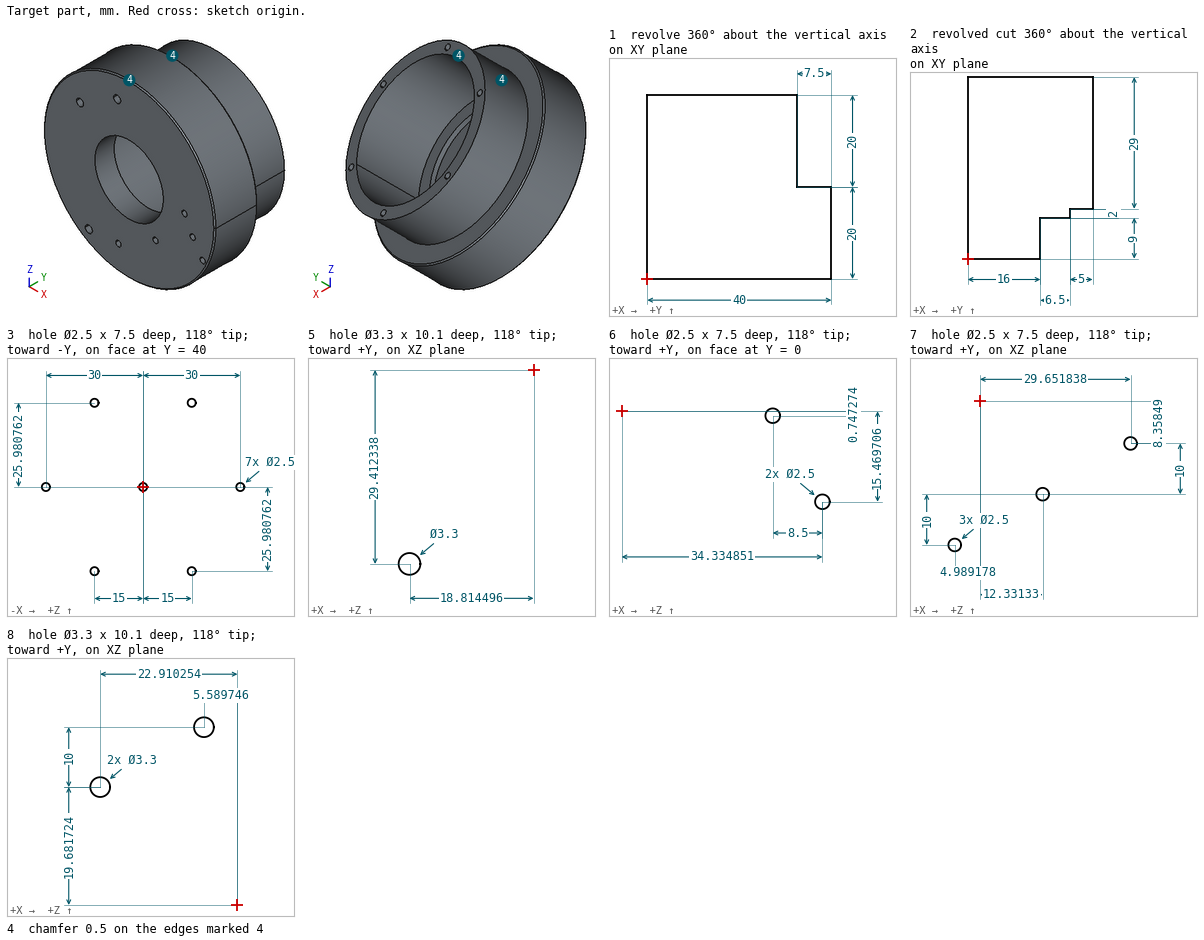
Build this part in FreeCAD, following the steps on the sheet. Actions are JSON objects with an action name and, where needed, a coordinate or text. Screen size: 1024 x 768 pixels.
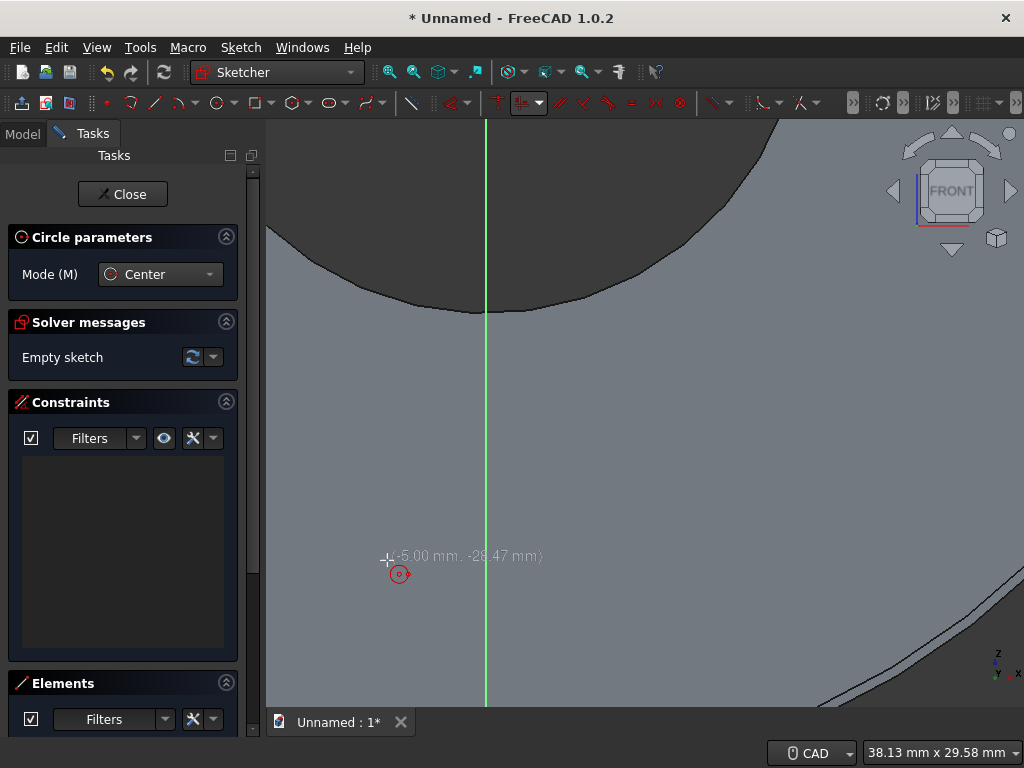
{"action": "left_click", "coordinate": [387, 559]}
{"action": "mouse_move", "coordinate": [405, 541]}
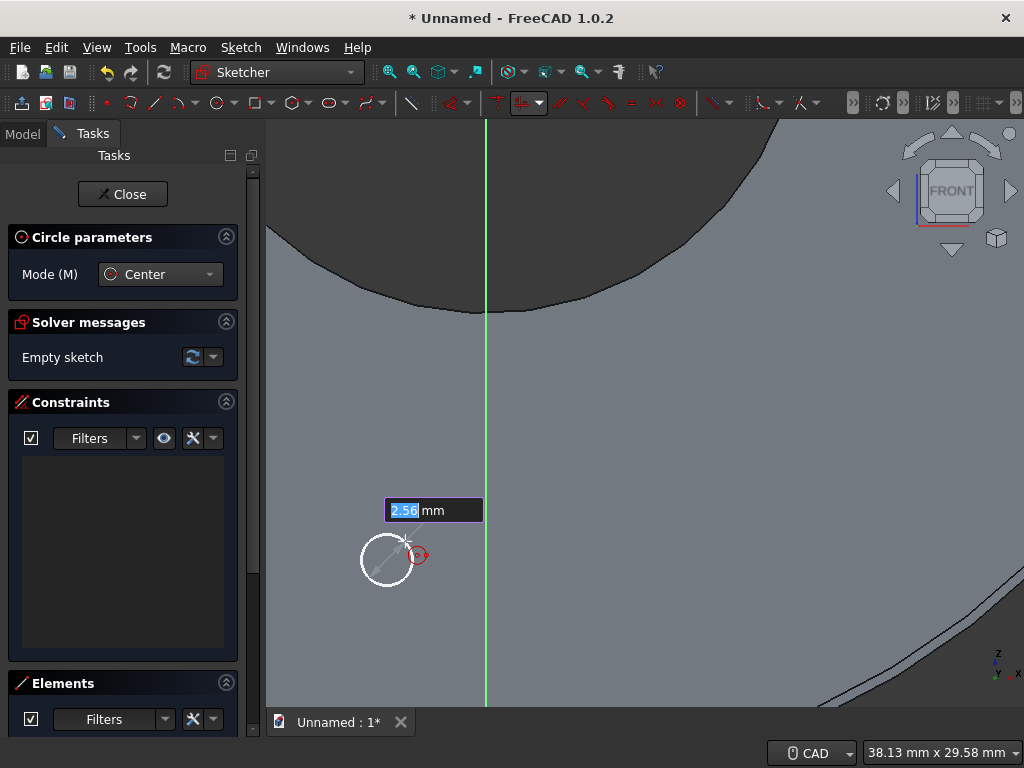
{"action": "type", "text": "2.5"}
{"action": "key", "text": "Return"}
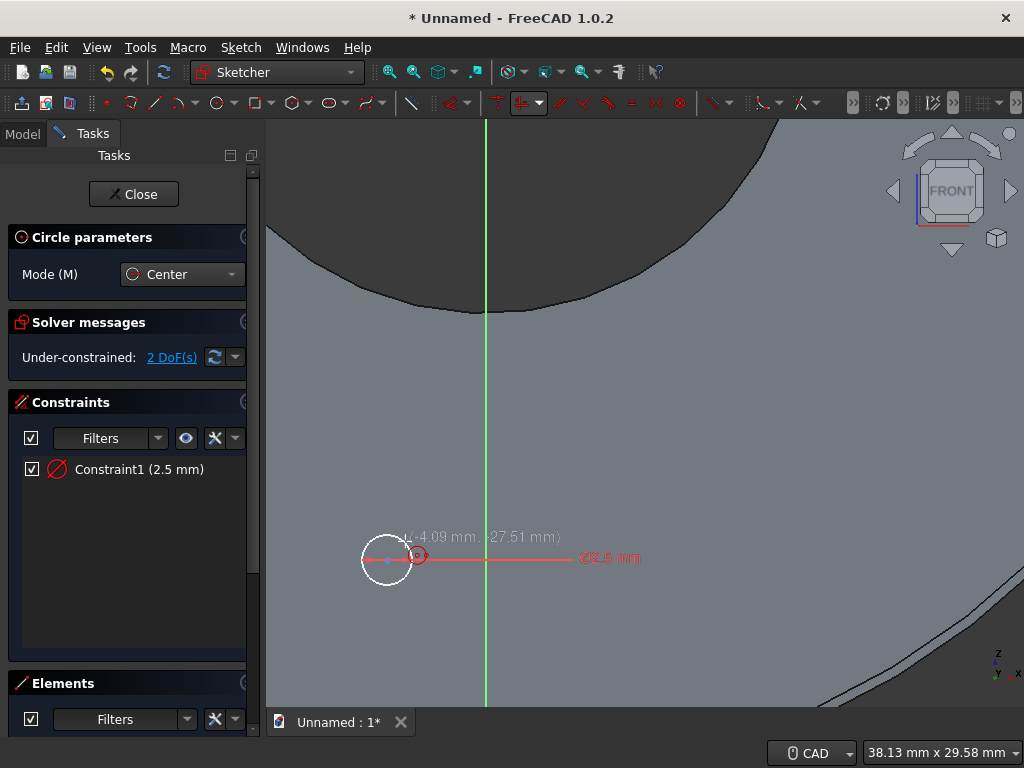
{"action": "left_click", "coordinate": [731, 360]}
{"action": "mouse_move", "coordinate": [749, 343]}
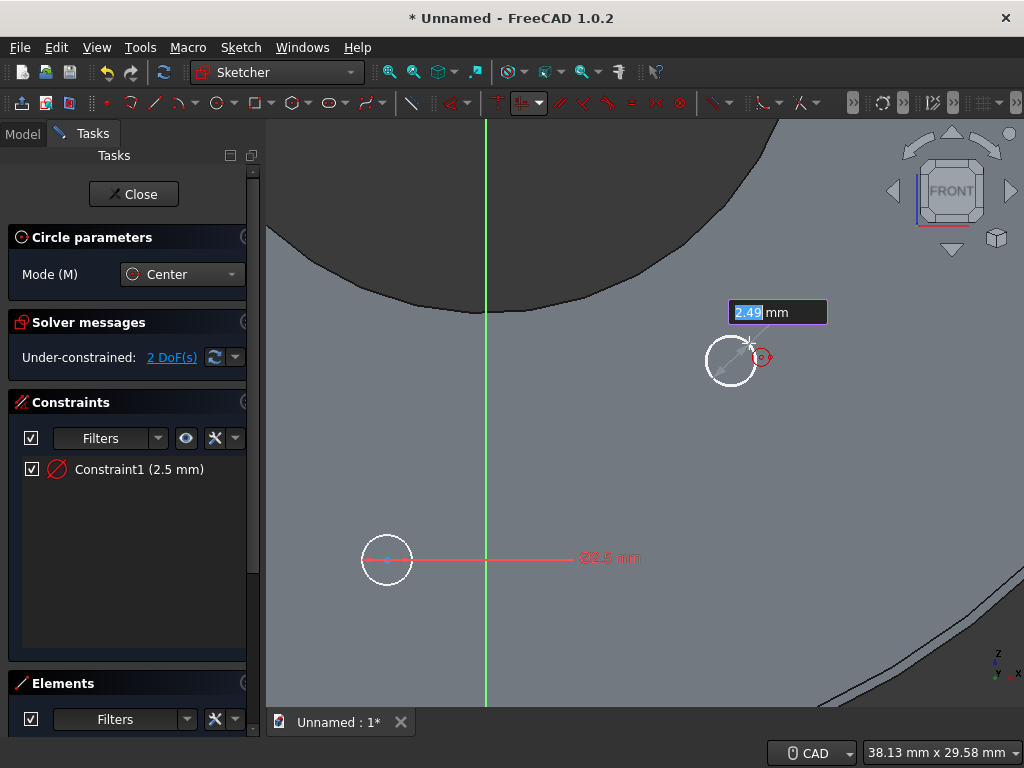
{"action": "type", "text": "2.5"}
{"action": "key", "text": "Return"}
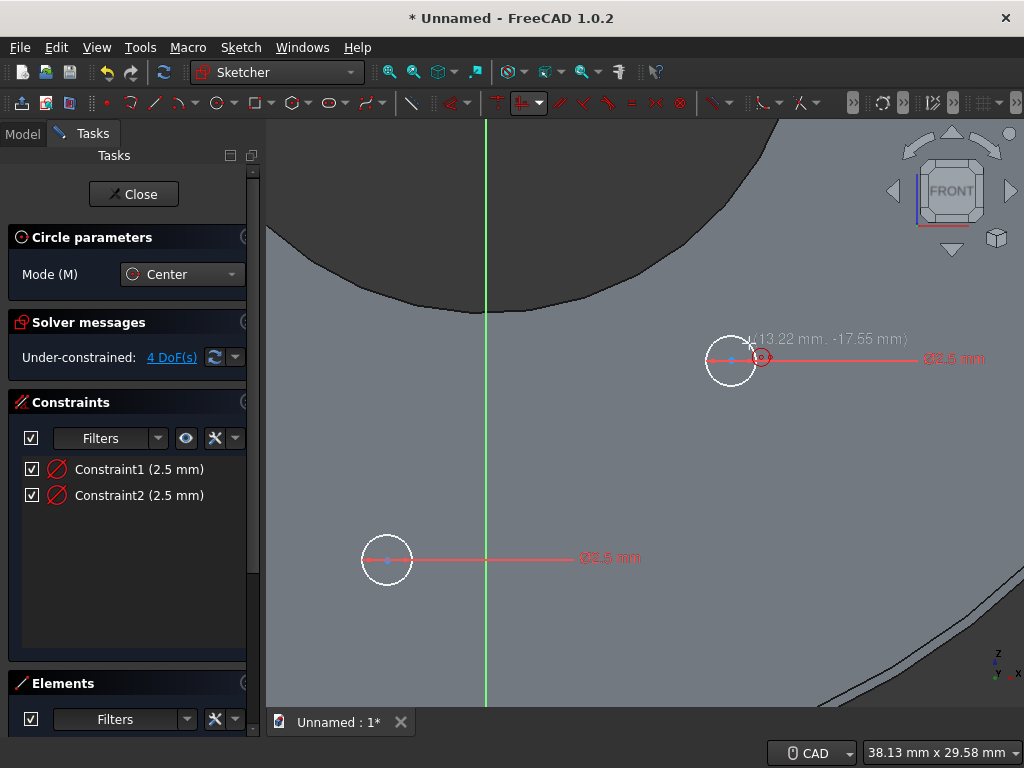
{"action": "scroll", "coordinate": [388, 563], "scroll_direction": "down", "scroll_amount": 3}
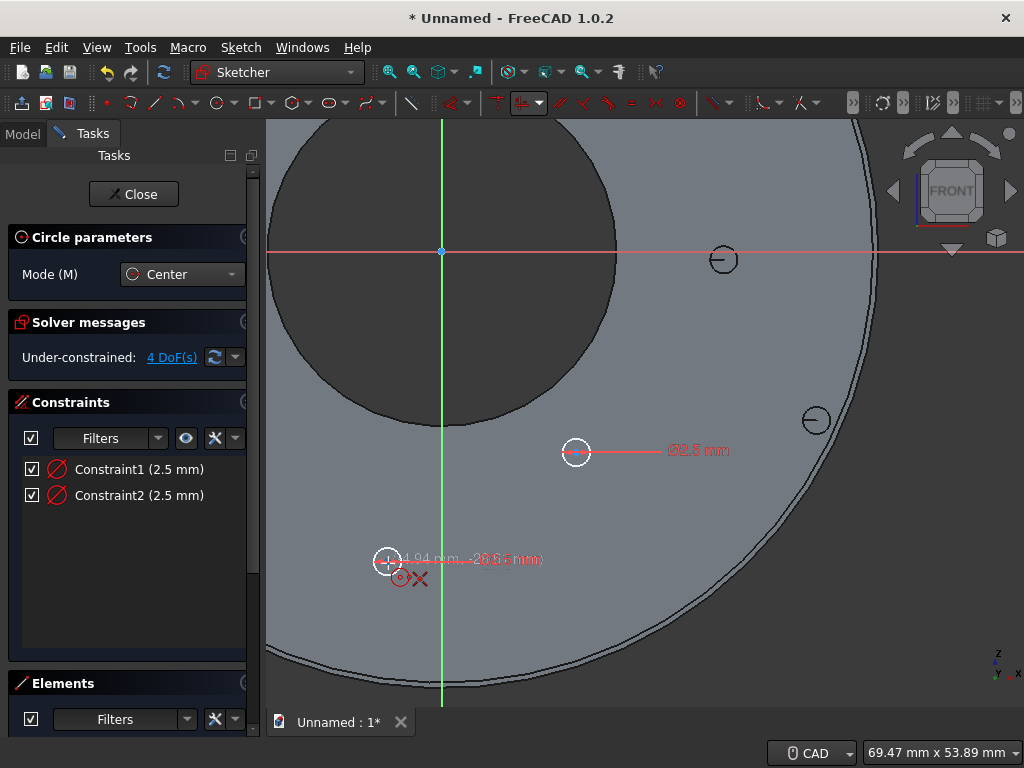
{"action": "scroll", "coordinate": [766, 343], "scroll_direction": "up", "scroll_amount": 3}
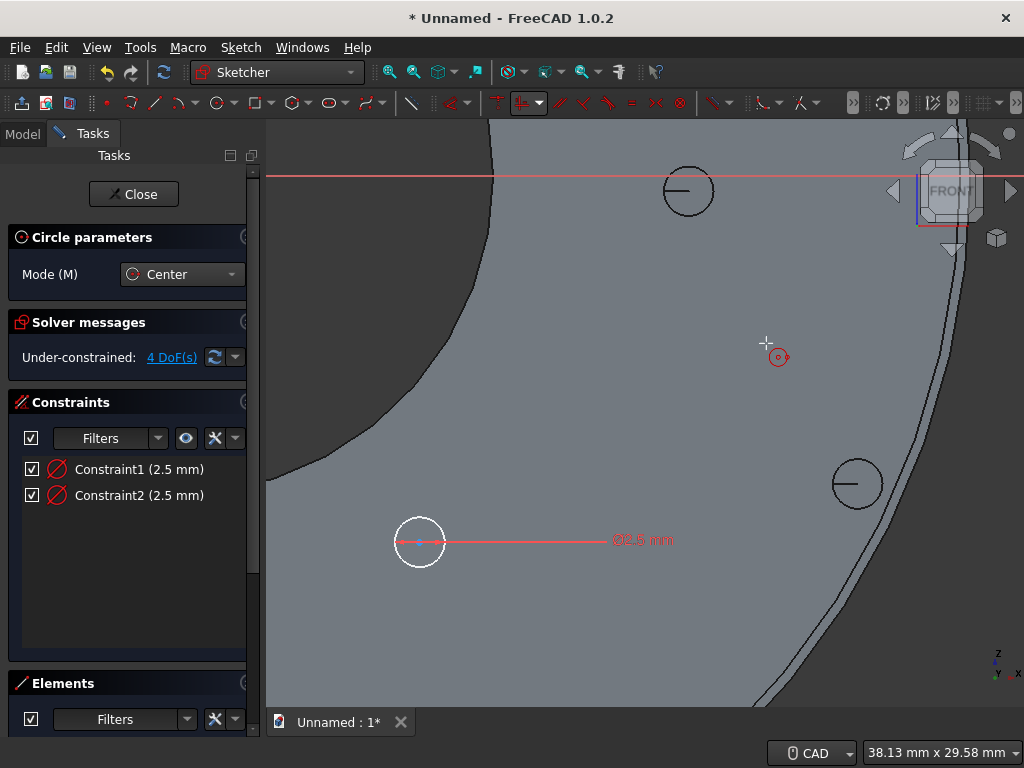
{"action": "left_click", "coordinate": [765, 343]}
{"action": "mouse_move", "coordinate": [782, 325]}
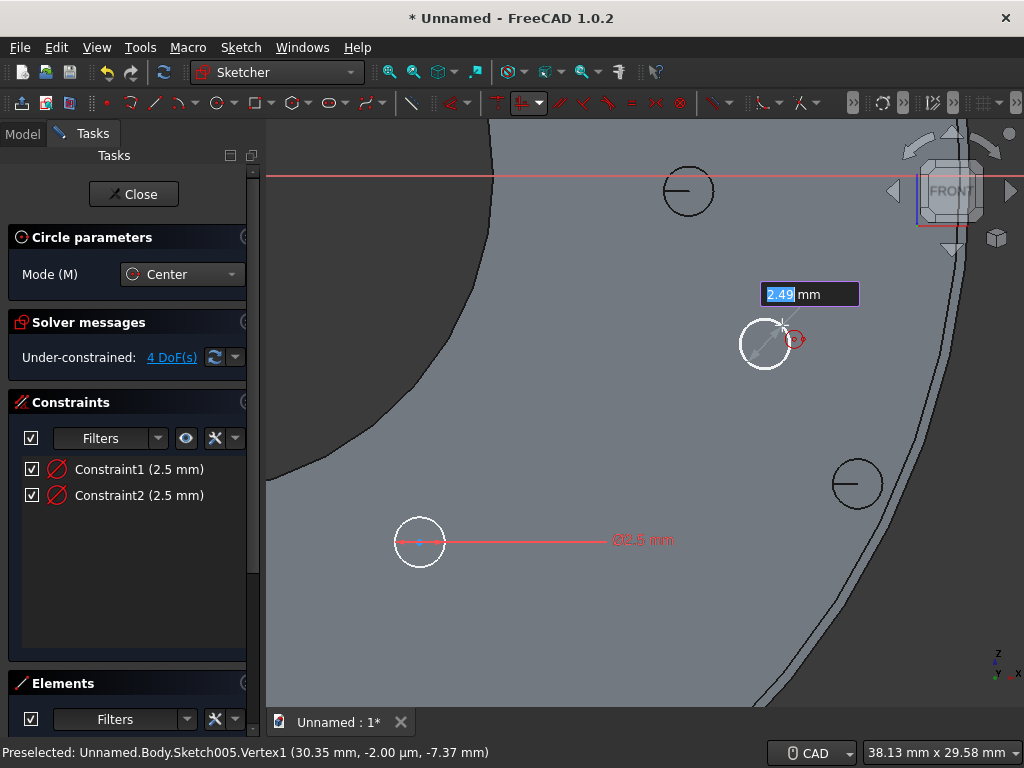
{"action": "type", "text": "2.5"}
{"action": "key", "text": "Return"}
{"action": "key", "text": "Escape"}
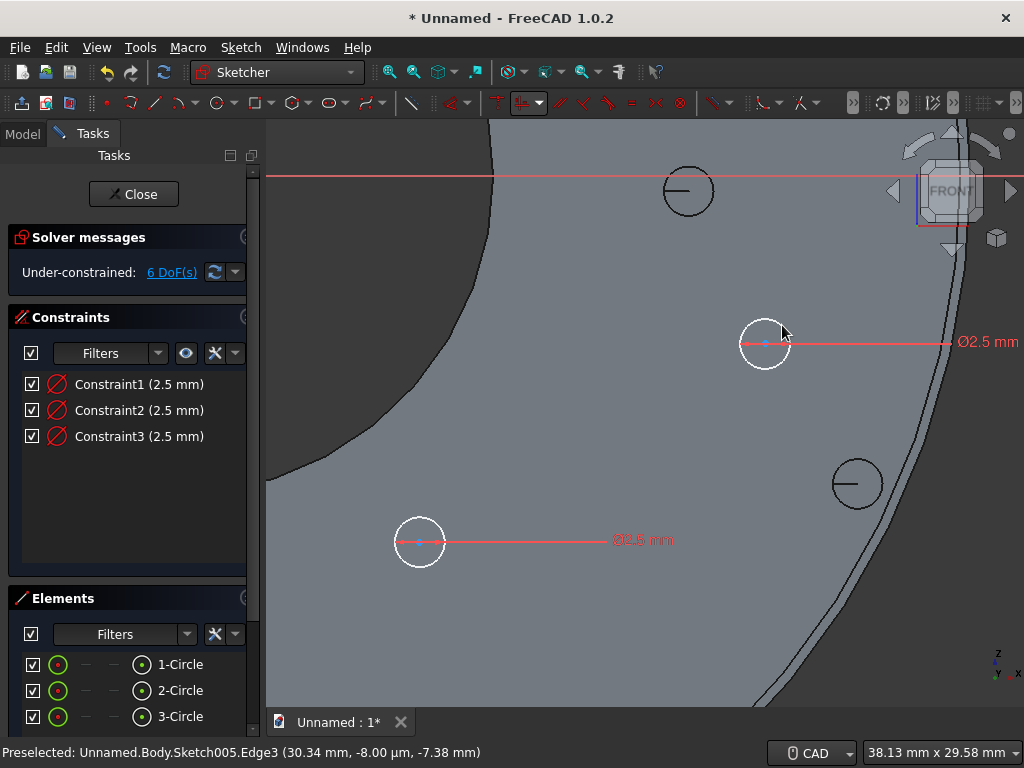
{"action": "left_click", "coordinate": [450, 104]}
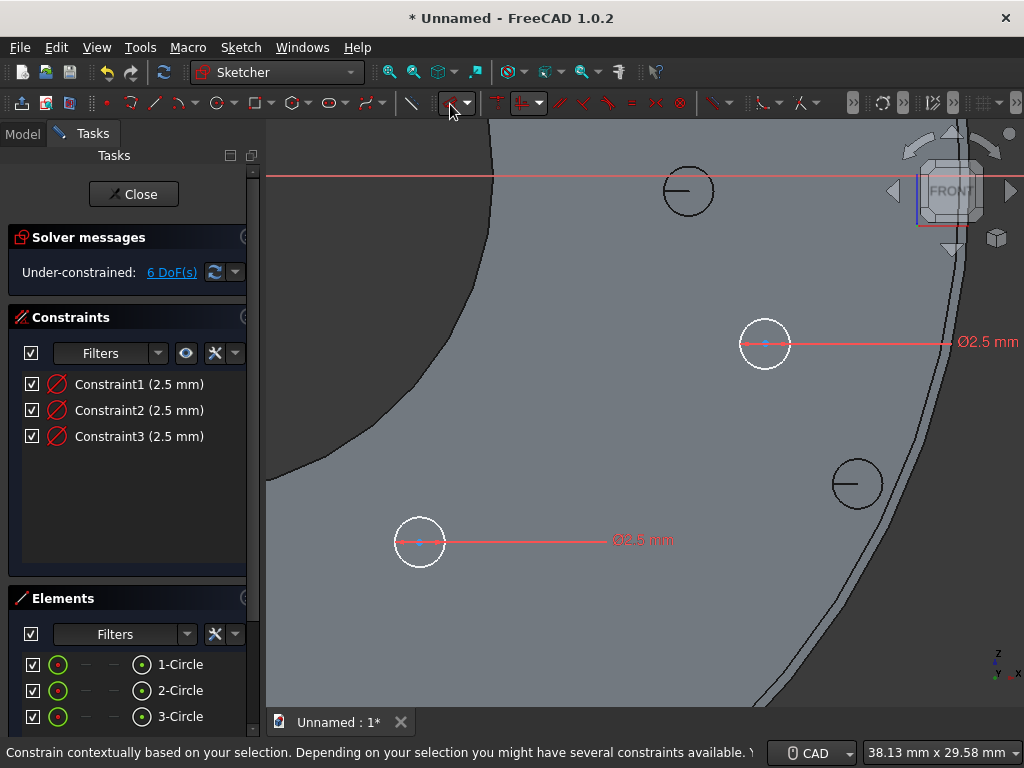
{"action": "scroll", "coordinate": [767, 343], "scroll_direction": "down", "scroll_amount": 3}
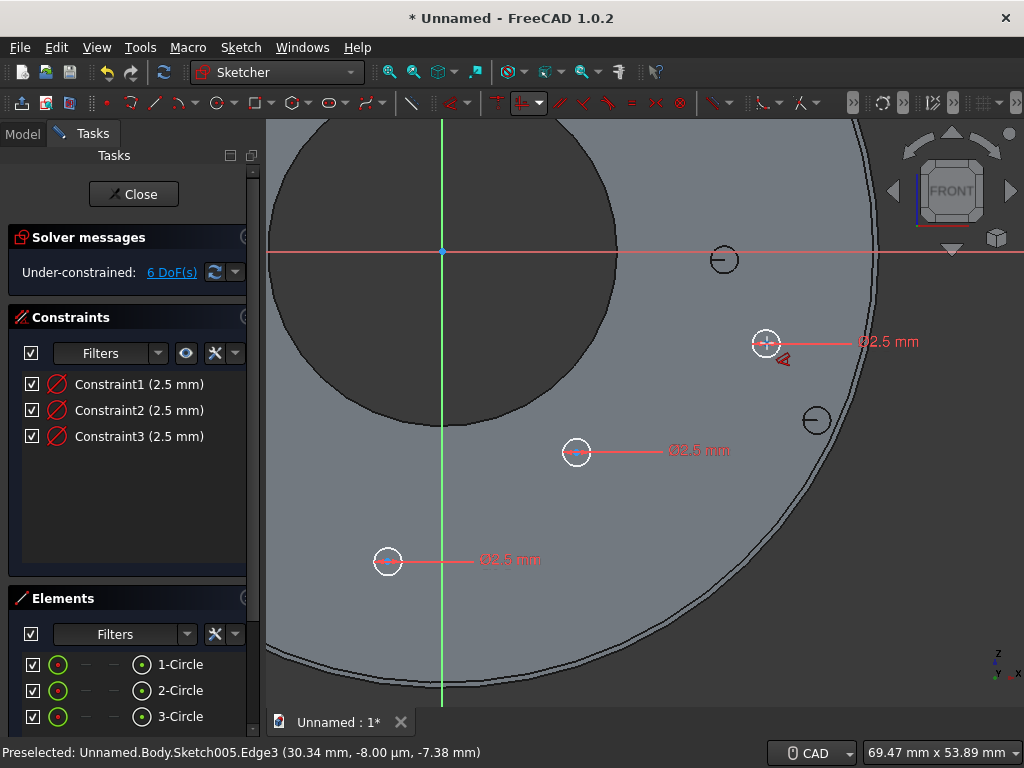
{"action": "left_click", "coordinate": [388, 562]}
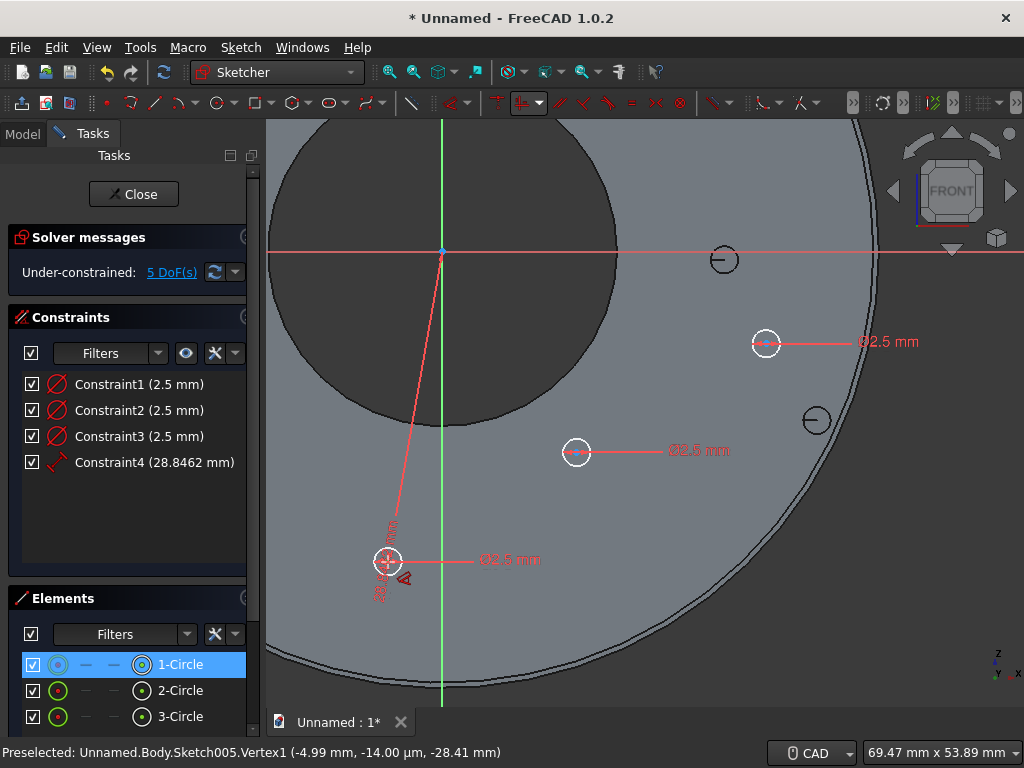
{"action": "left_click", "coordinate": [577, 452]}
{"action": "left_click", "coordinate": [354, 507]}